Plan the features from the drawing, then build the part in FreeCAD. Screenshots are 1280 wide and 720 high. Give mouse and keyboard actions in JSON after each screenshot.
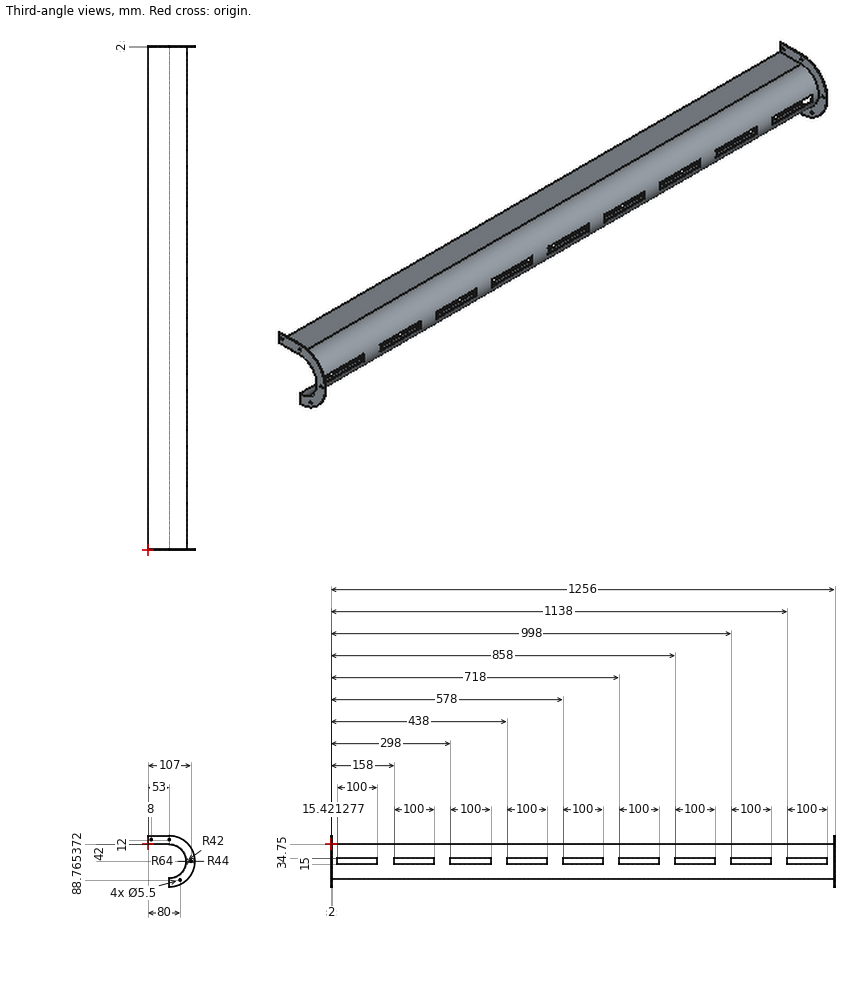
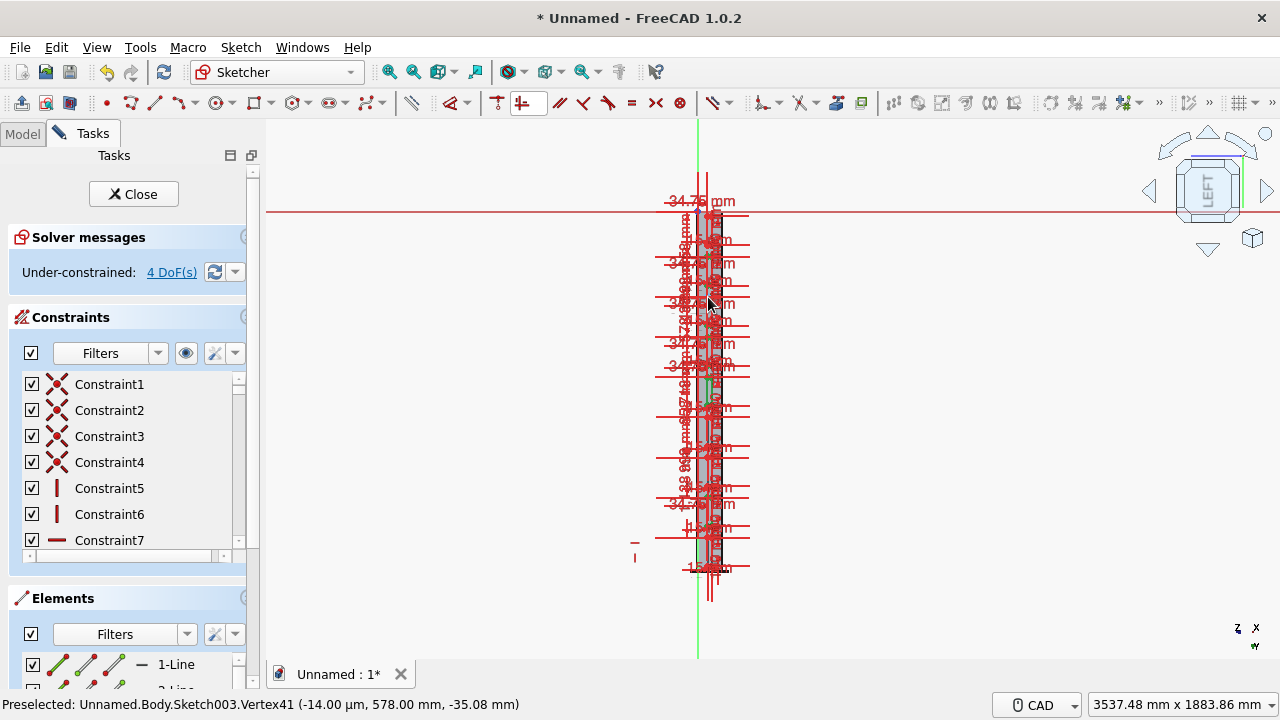
{"action": "scroll", "coordinate": [708, 417], "scroll_direction": "up", "scroll_amount": 7}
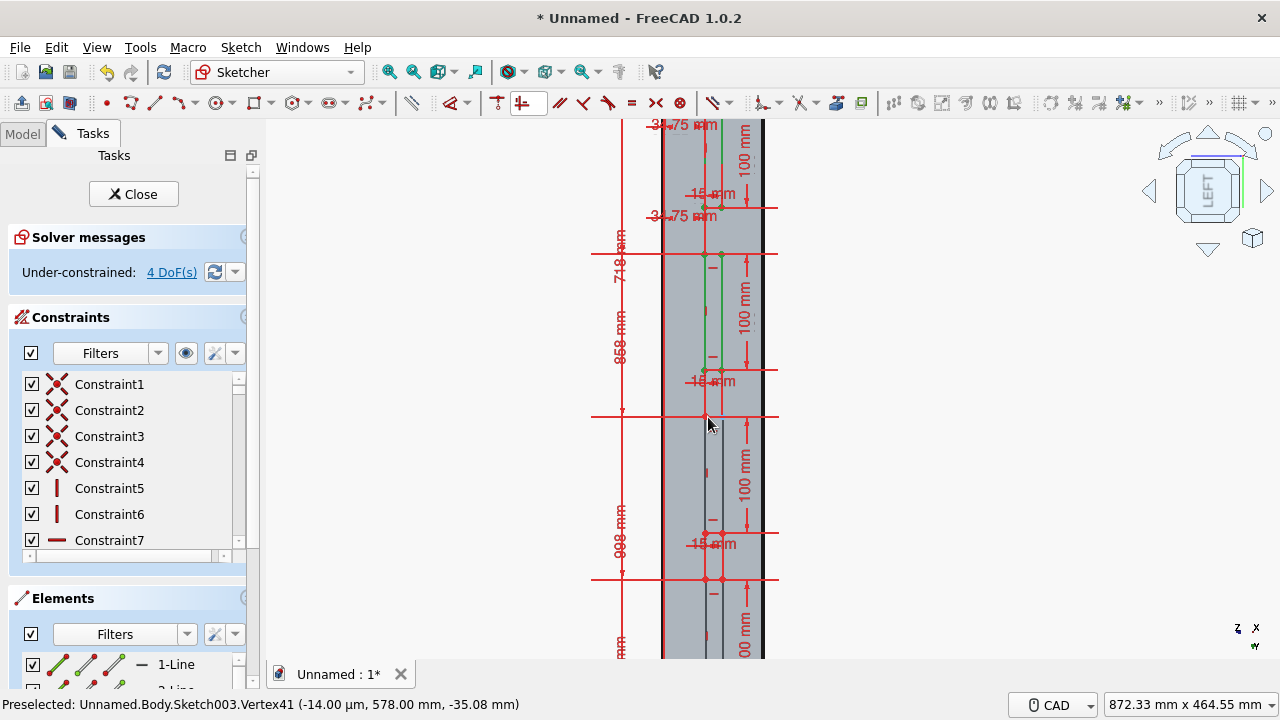
{"action": "left_click", "coordinate": [705, 417]}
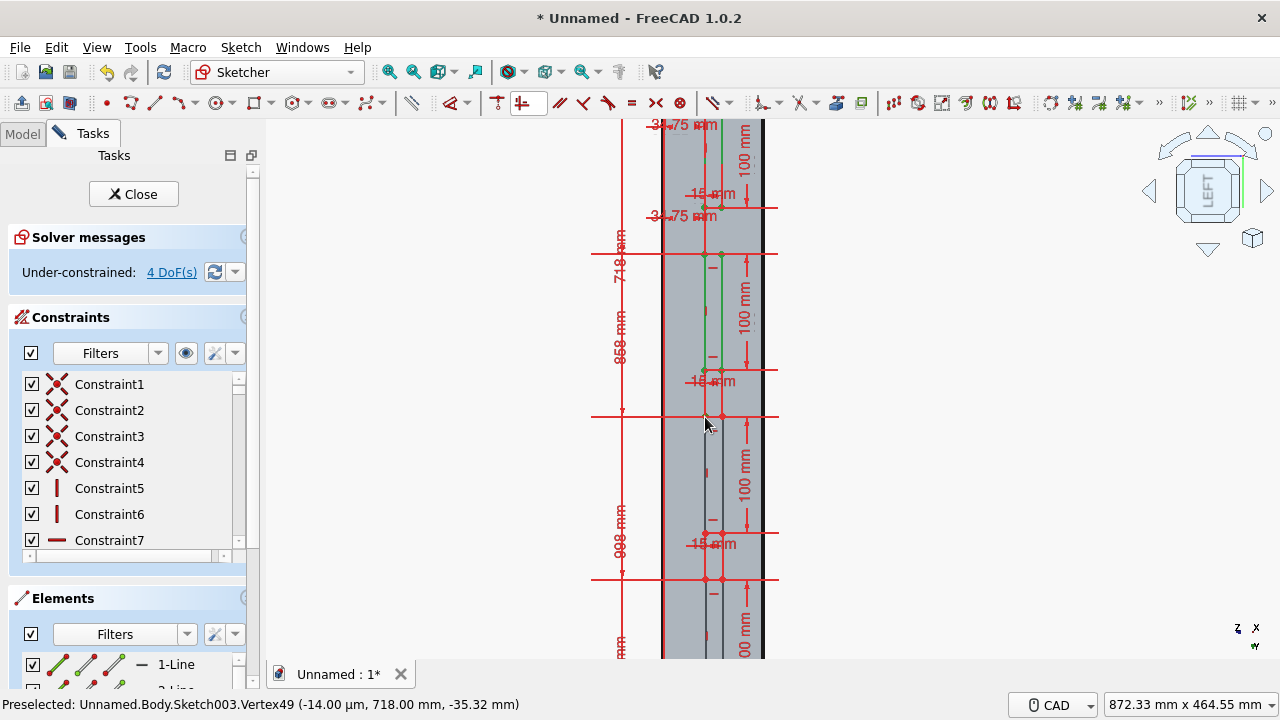
{"action": "key", "text": "l"}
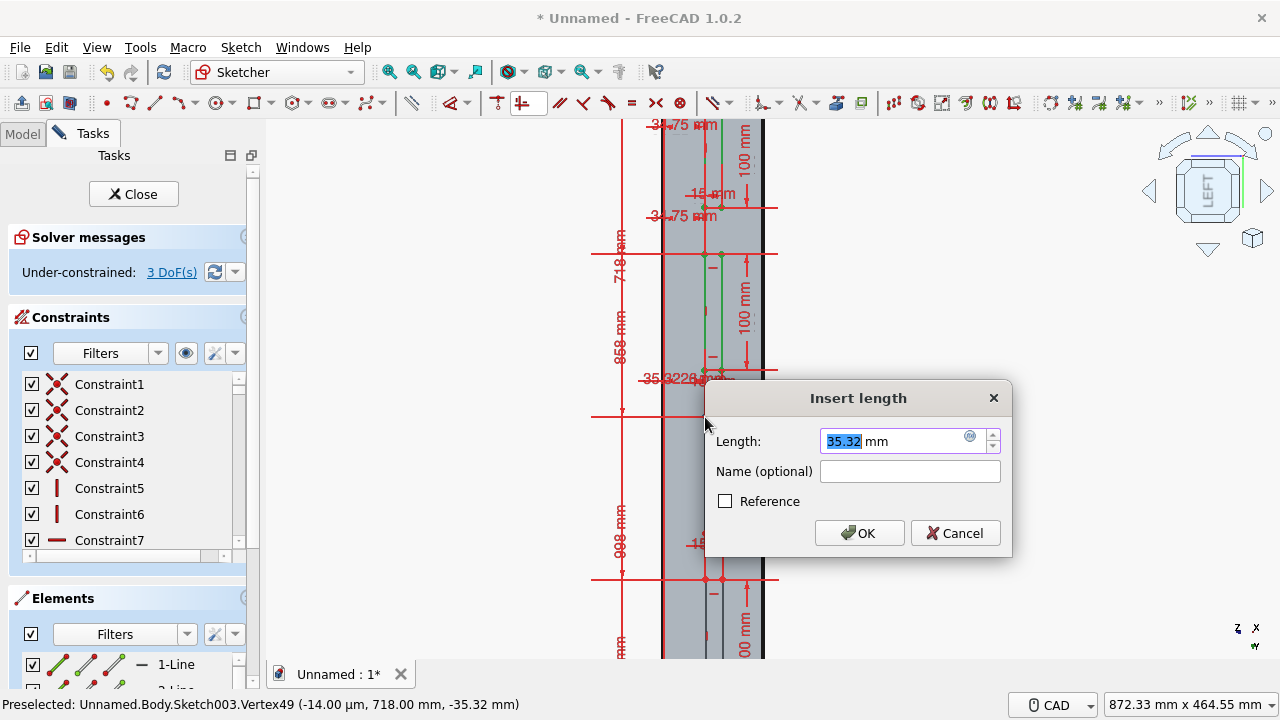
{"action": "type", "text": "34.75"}
{"action": "key", "text": "Return"}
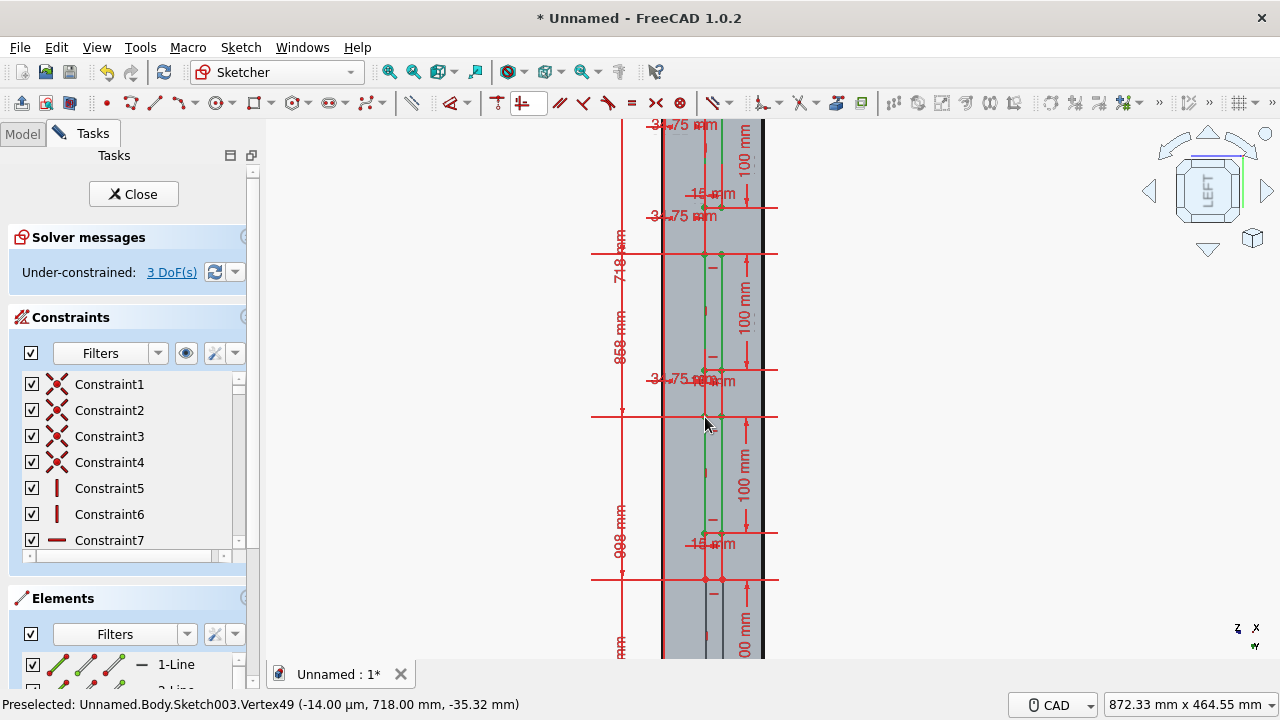
{"action": "left_click", "coordinate": [706, 580]}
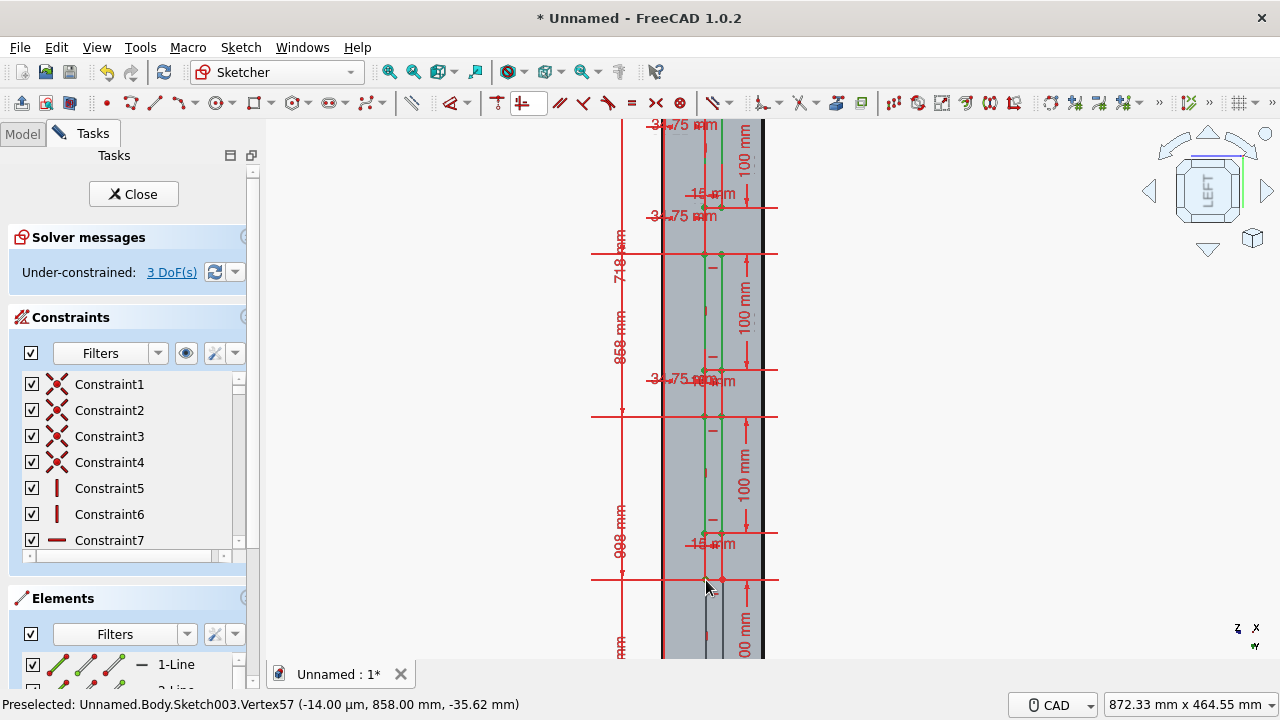
{"action": "left_click", "coordinate": [470, 104]}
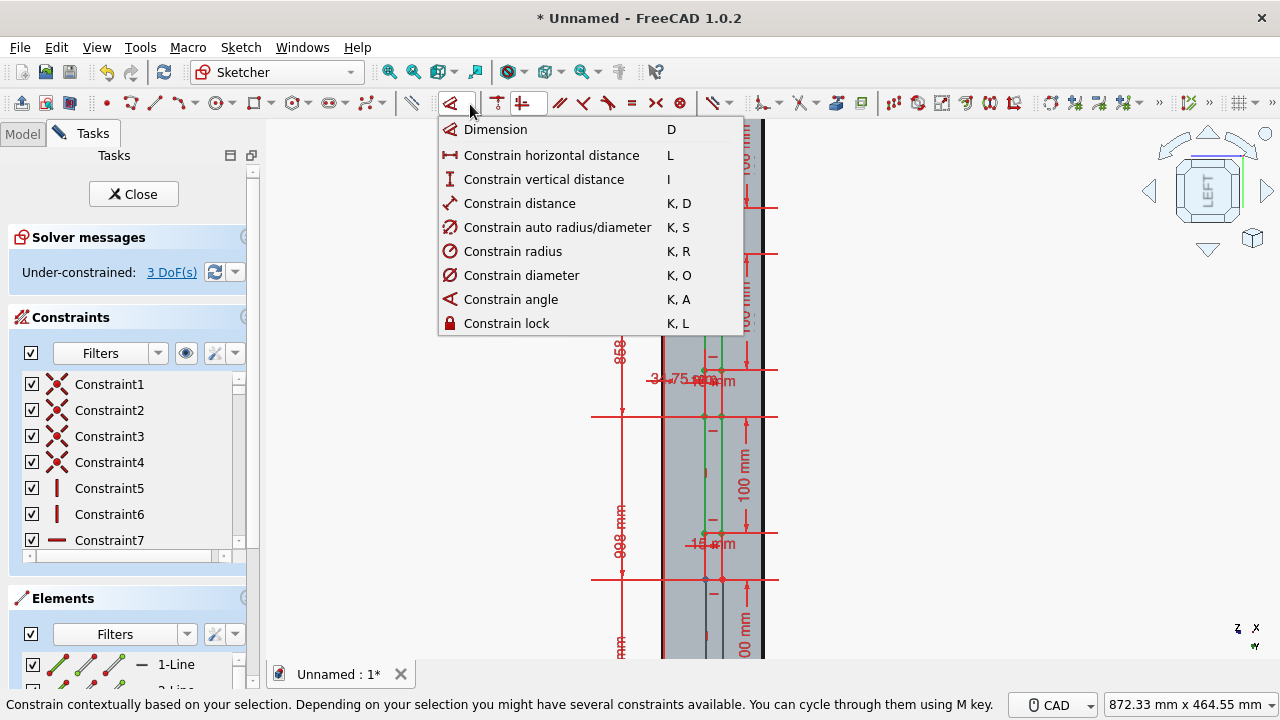
{"action": "left_click", "coordinate": [591, 155]}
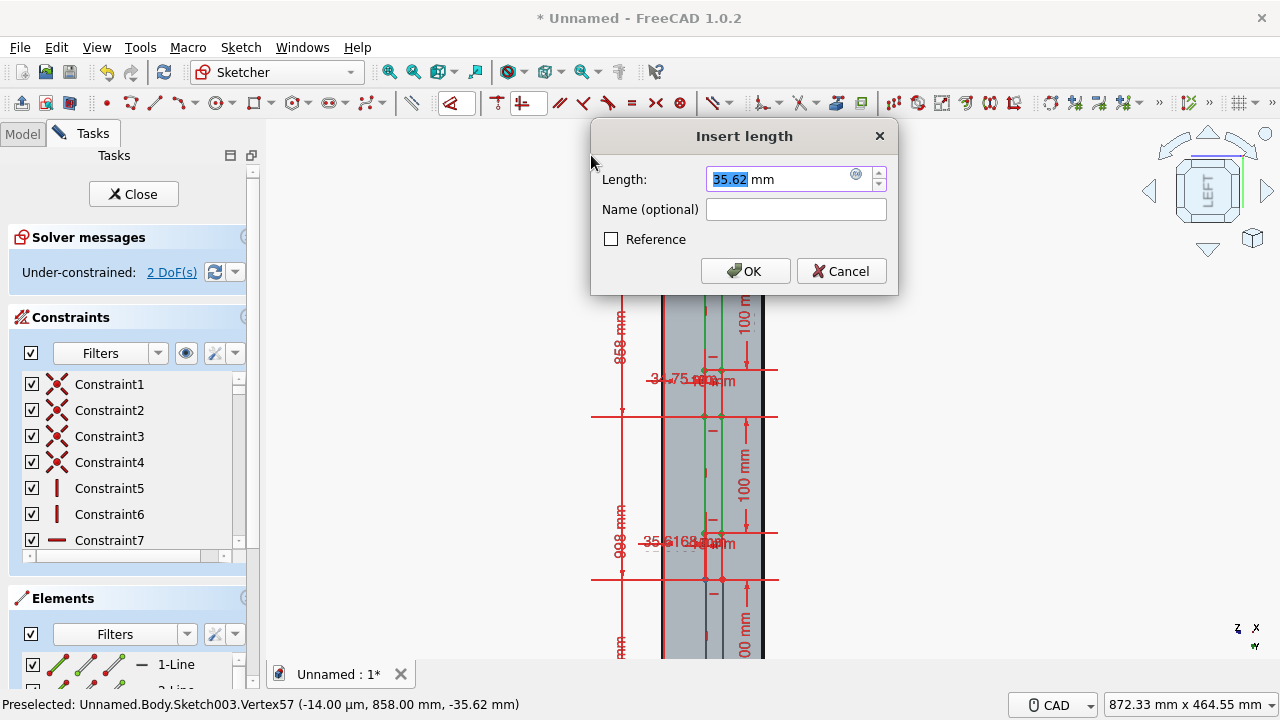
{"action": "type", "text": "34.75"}
{"action": "key", "text": "Return"}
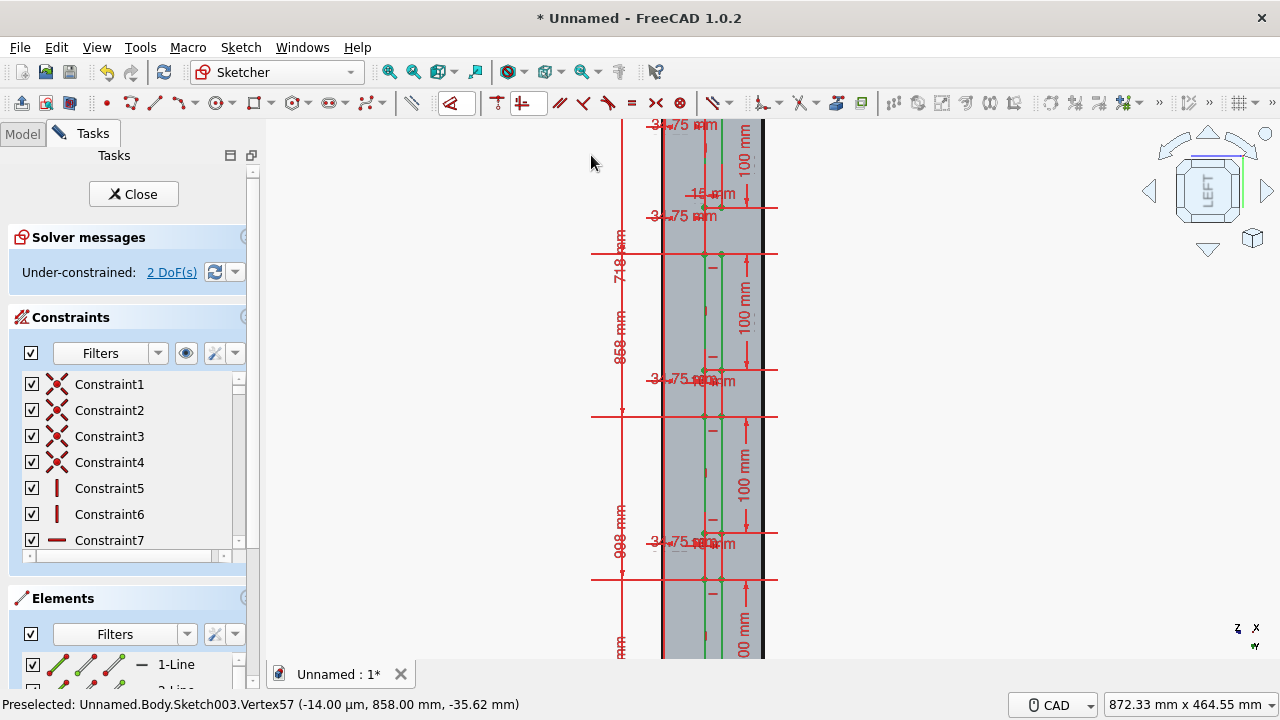
{"action": "scroll", "coordinate": [708, 418], "scroll_direction": "down", "scroll_amount": 7}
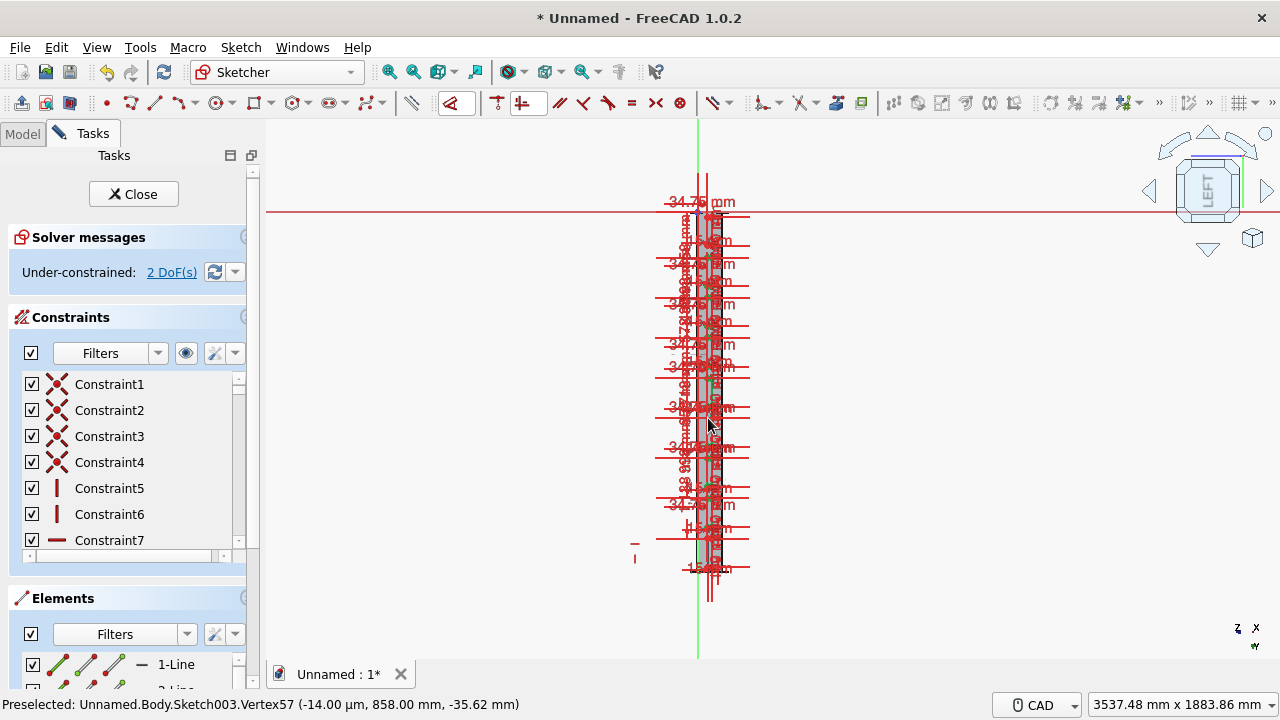
{"action": "scroll", "coordinate": [708, 539], "scroll_direction": "up", "scroll_amount": 7}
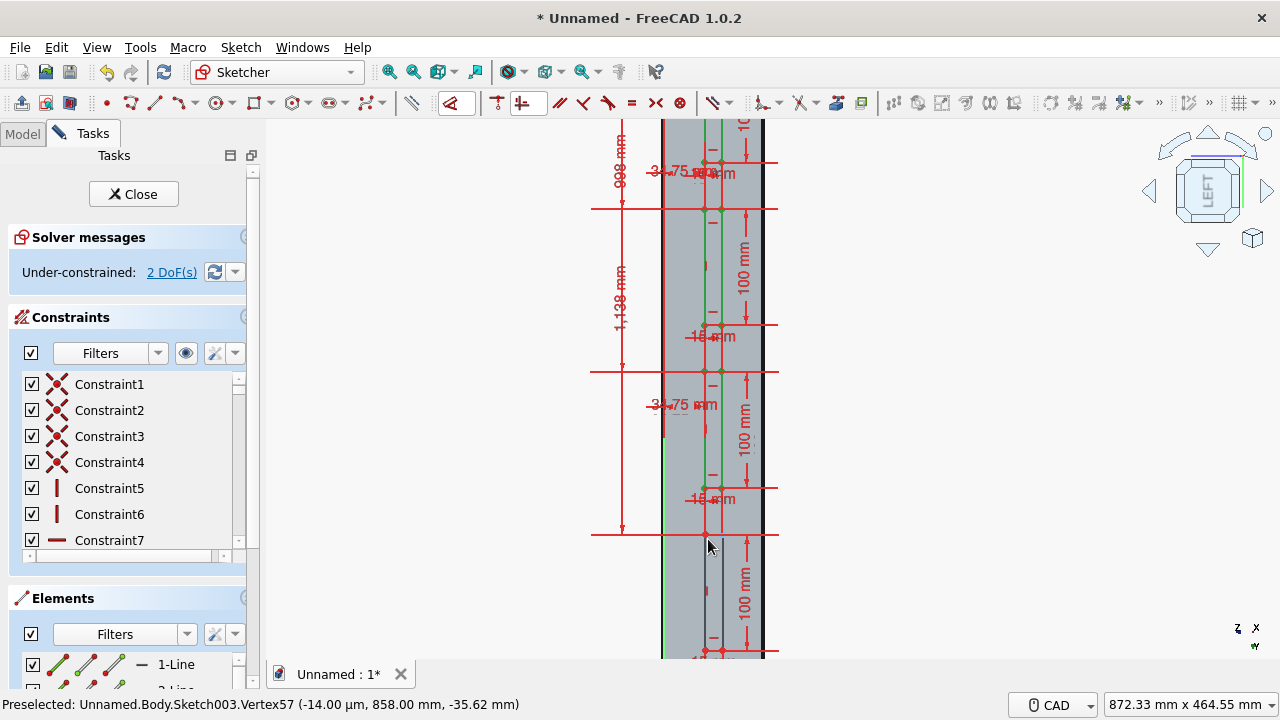
{"action": "left_click", "coordinate": [705, 535]}